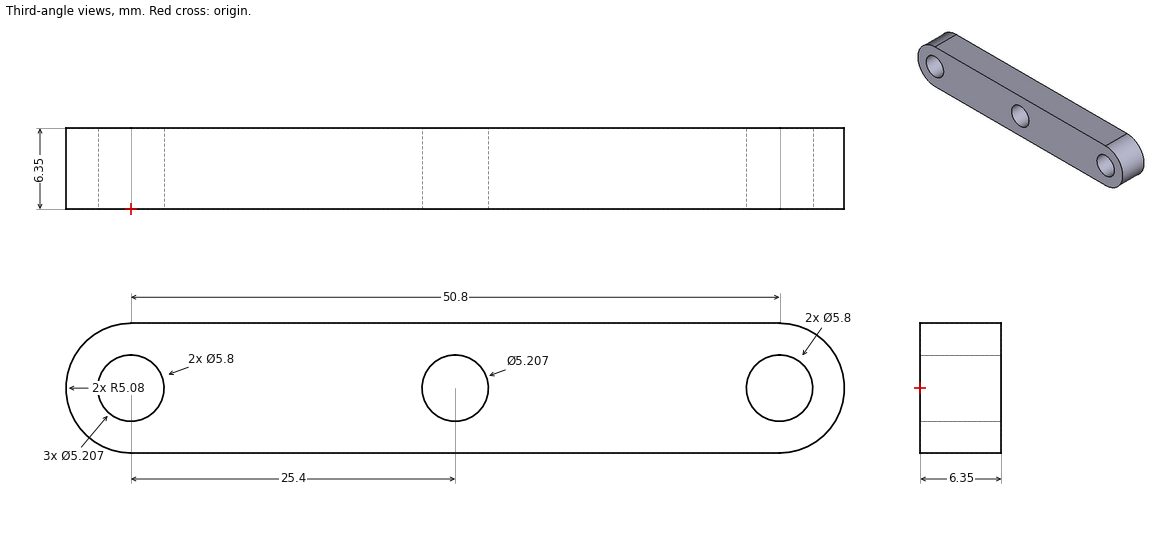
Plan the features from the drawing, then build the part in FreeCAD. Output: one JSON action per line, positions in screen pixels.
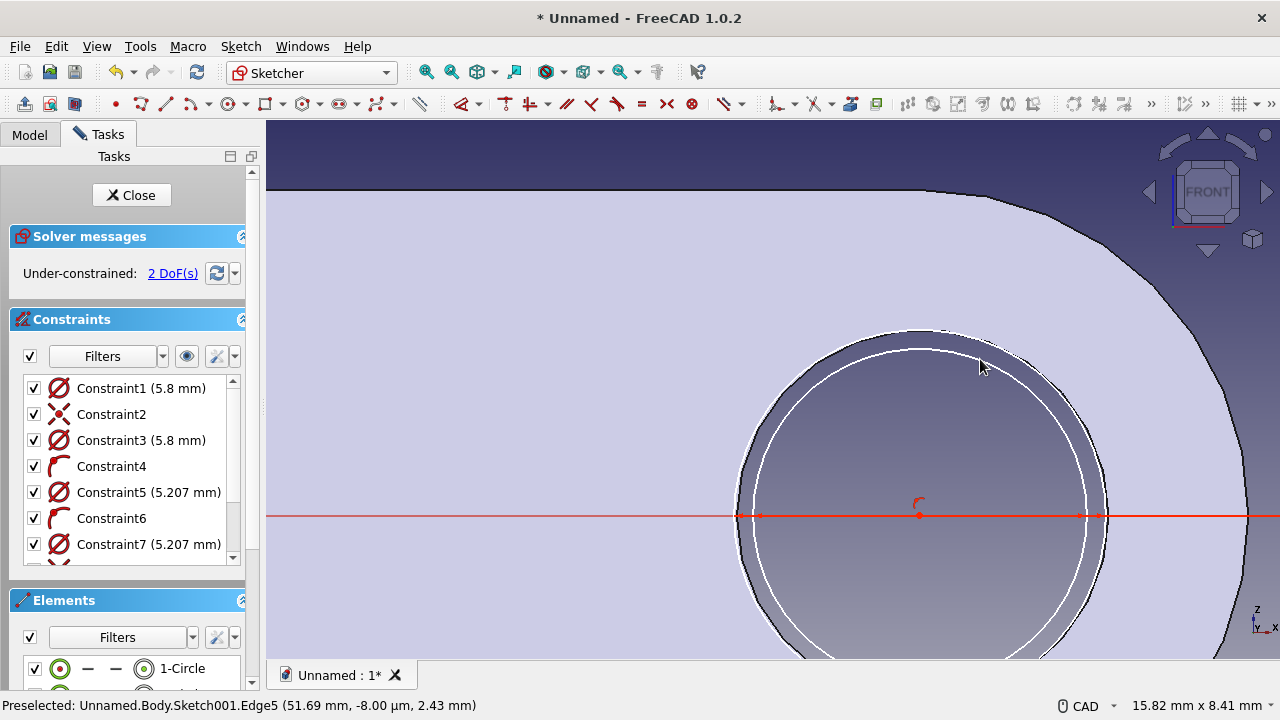
{"action": "key", "text": "d"}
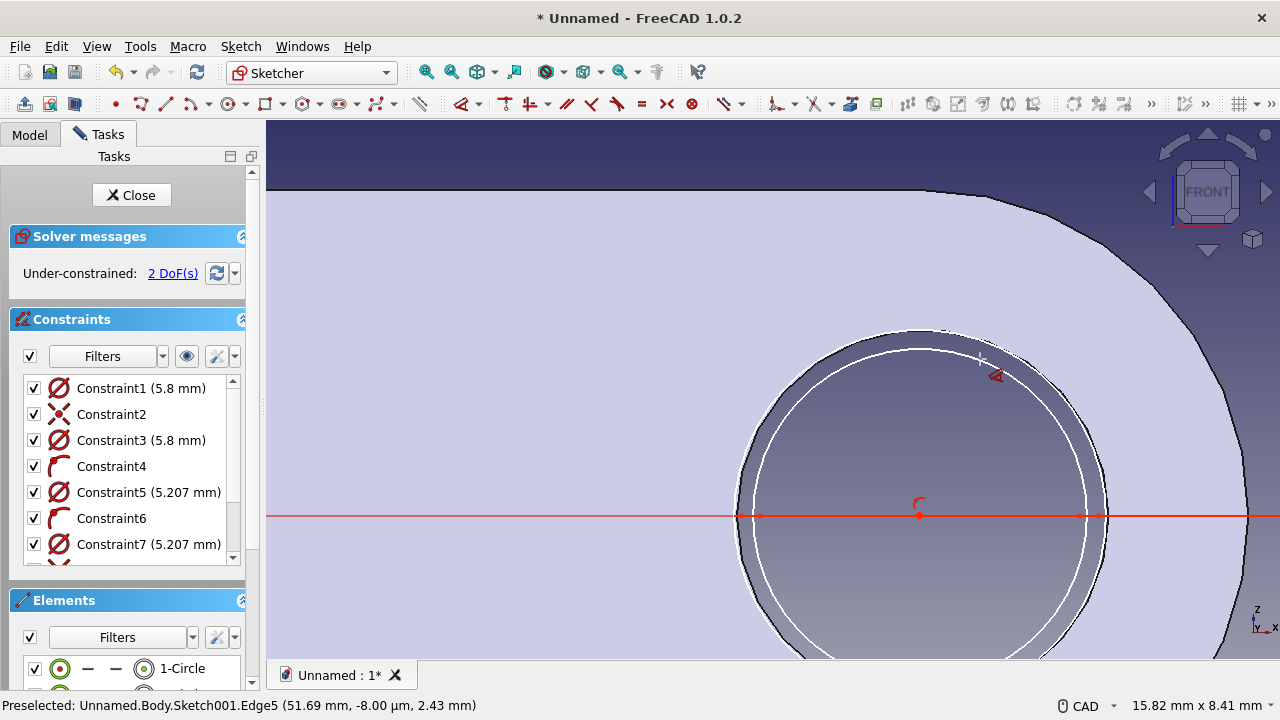
{"action": "scroll", "coordinate": [984, 364], "scroll_direction": "down", "scroll_amount": 9}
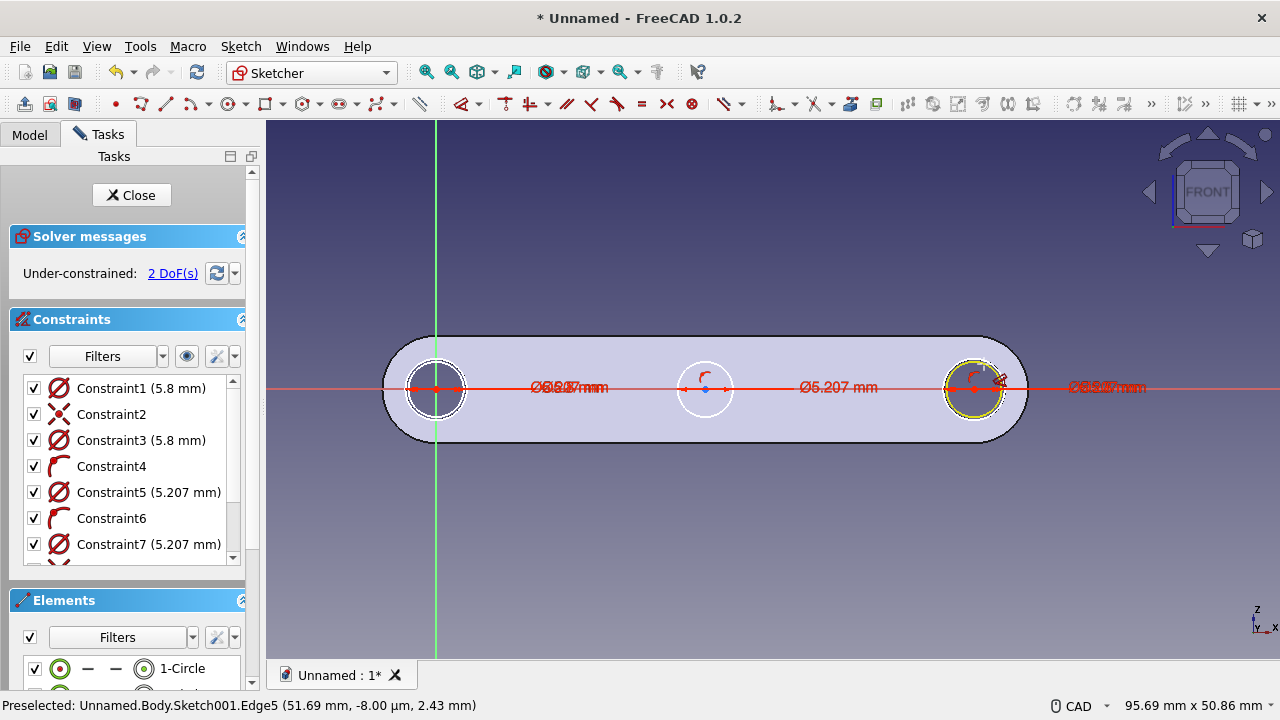
{"action": "left_click", "coordinate": [974, 389]}
{"action": "left_click", "coordinate": [581, 423]}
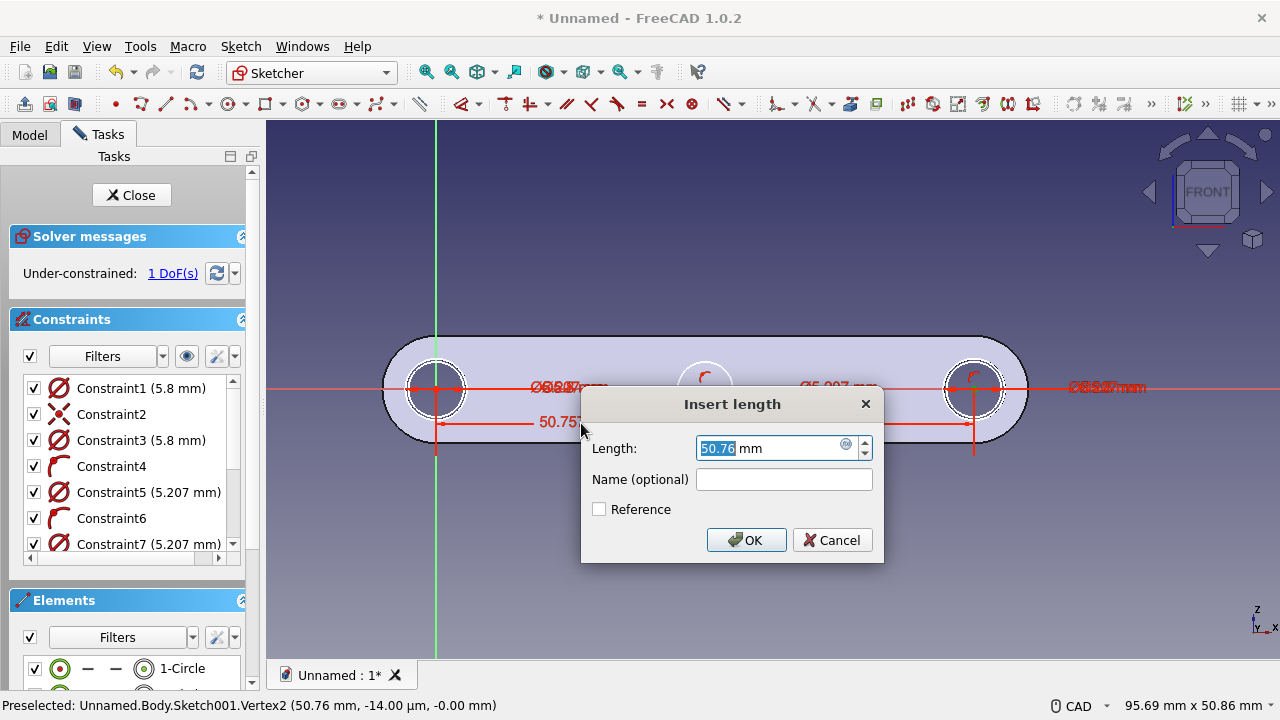
{"action": "type", "text": "50.8"}
{"action": "key", "text": "Return"}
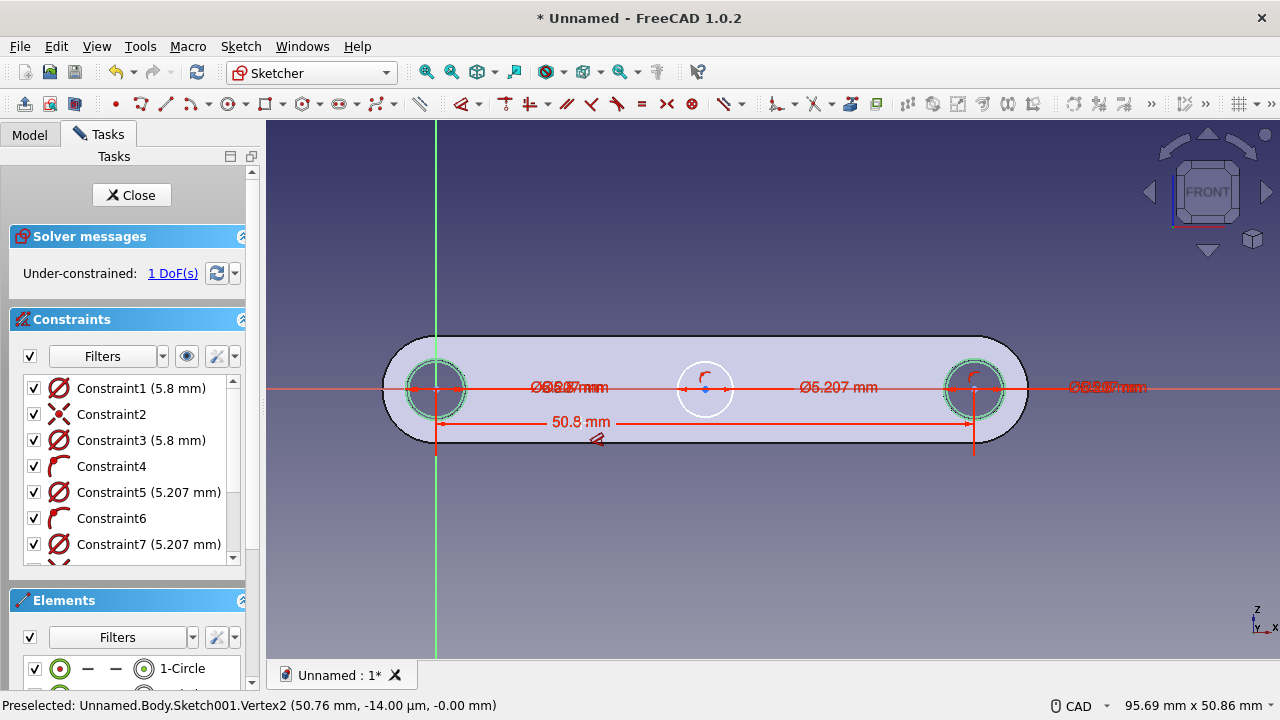
{"action": "left_click", "coordinate": [705, 389]}
{"action": "left_click", "coordinate": [509, 423]}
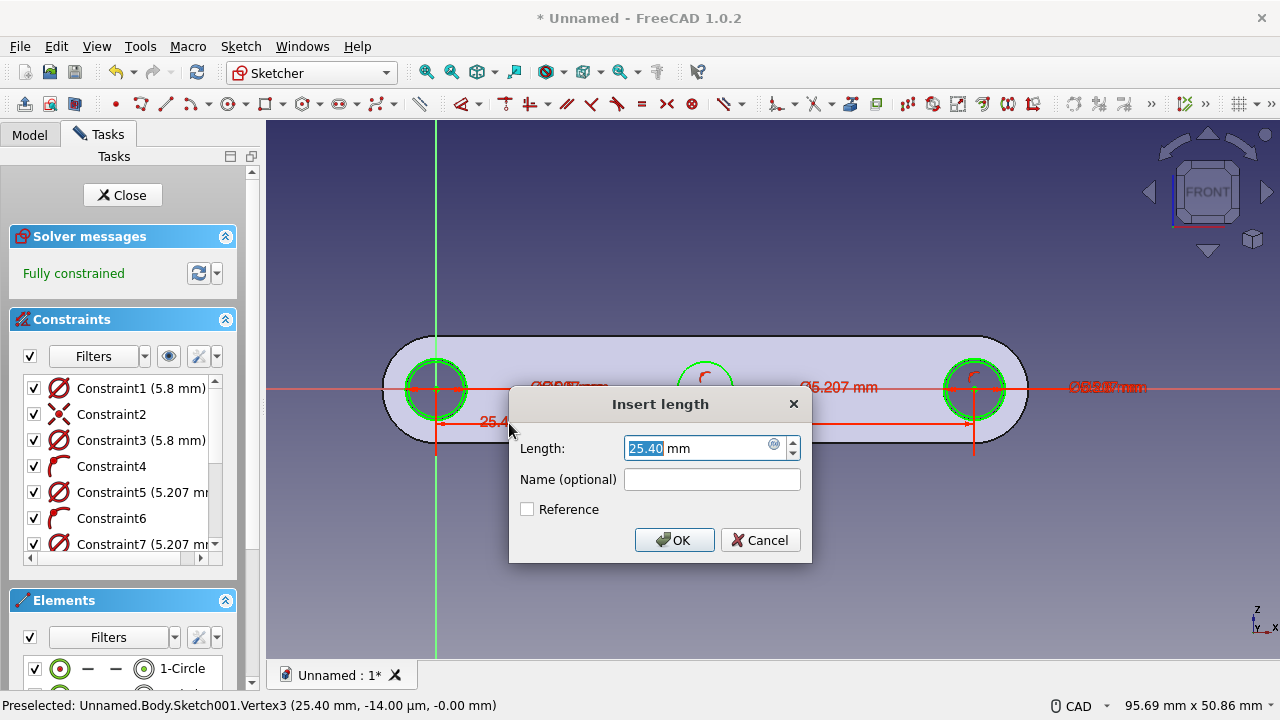
{"action": "type", "text": "25.4"}
{"action": "key", "text": "Return"}
{"action": "key", "text": "Escape"}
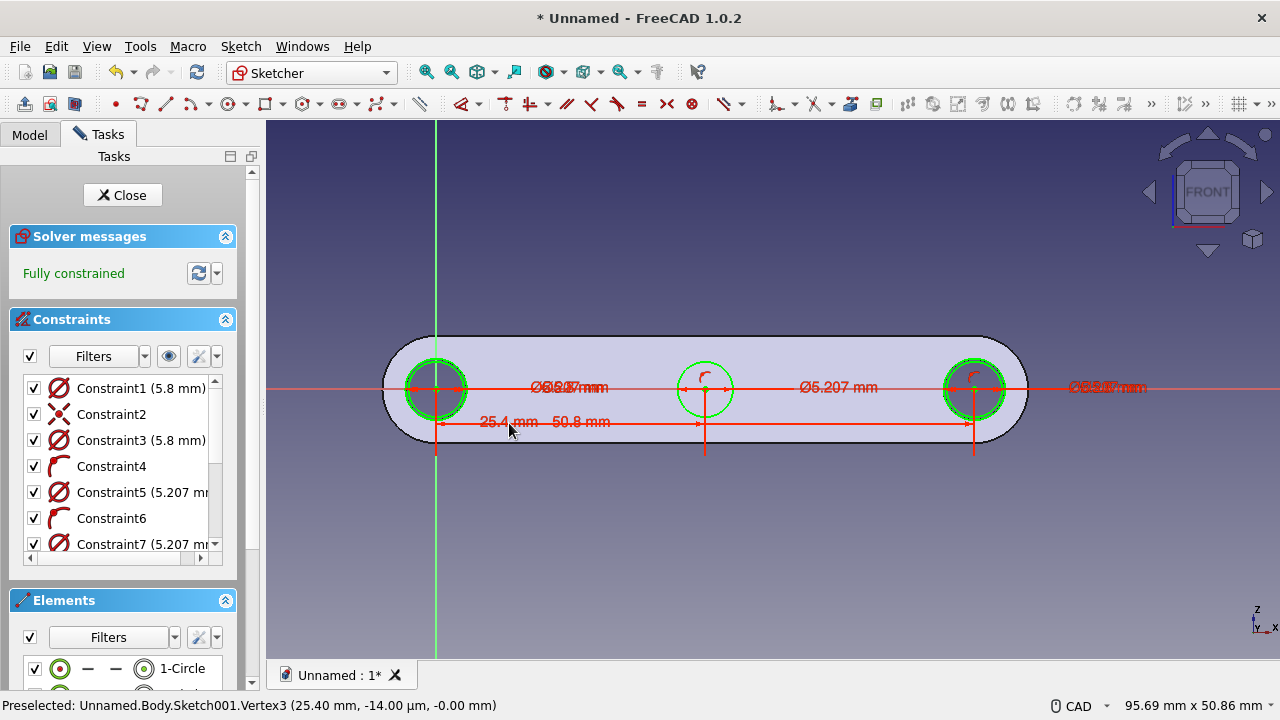
{"action": "left_click", "coordinate": [123, 195]}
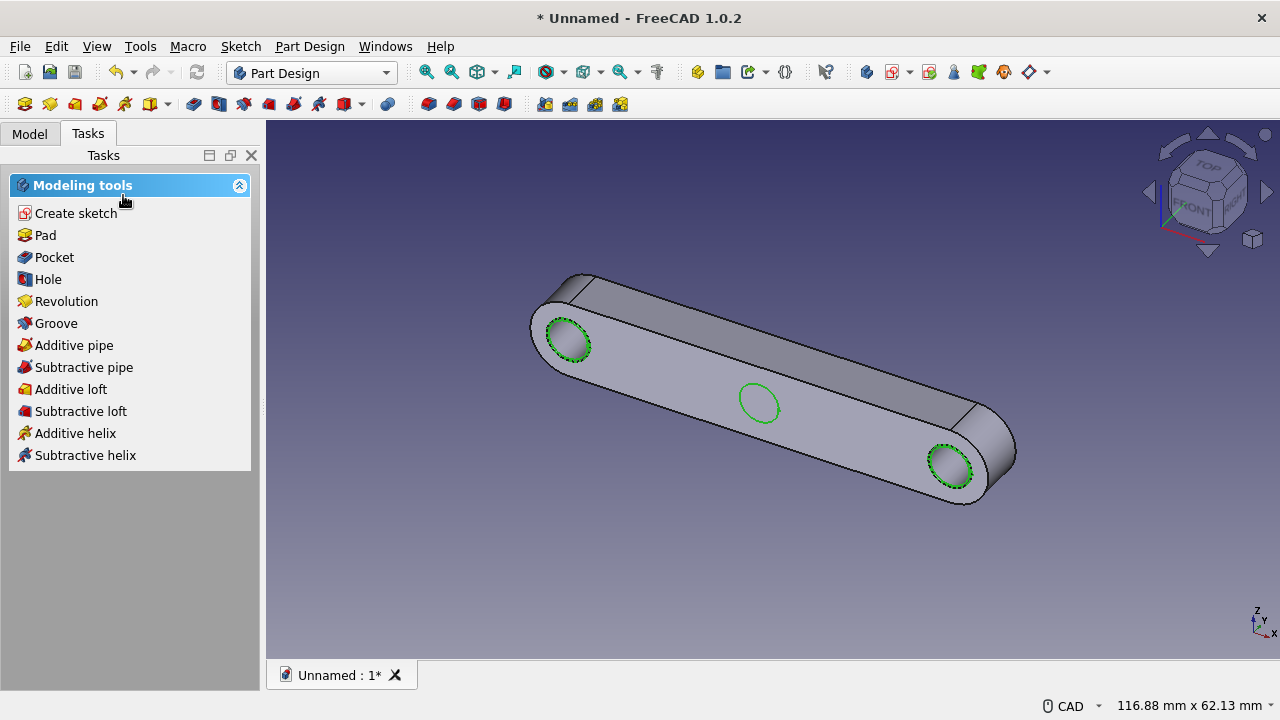
{"action": "left_click", "coordinate": [25, 104]}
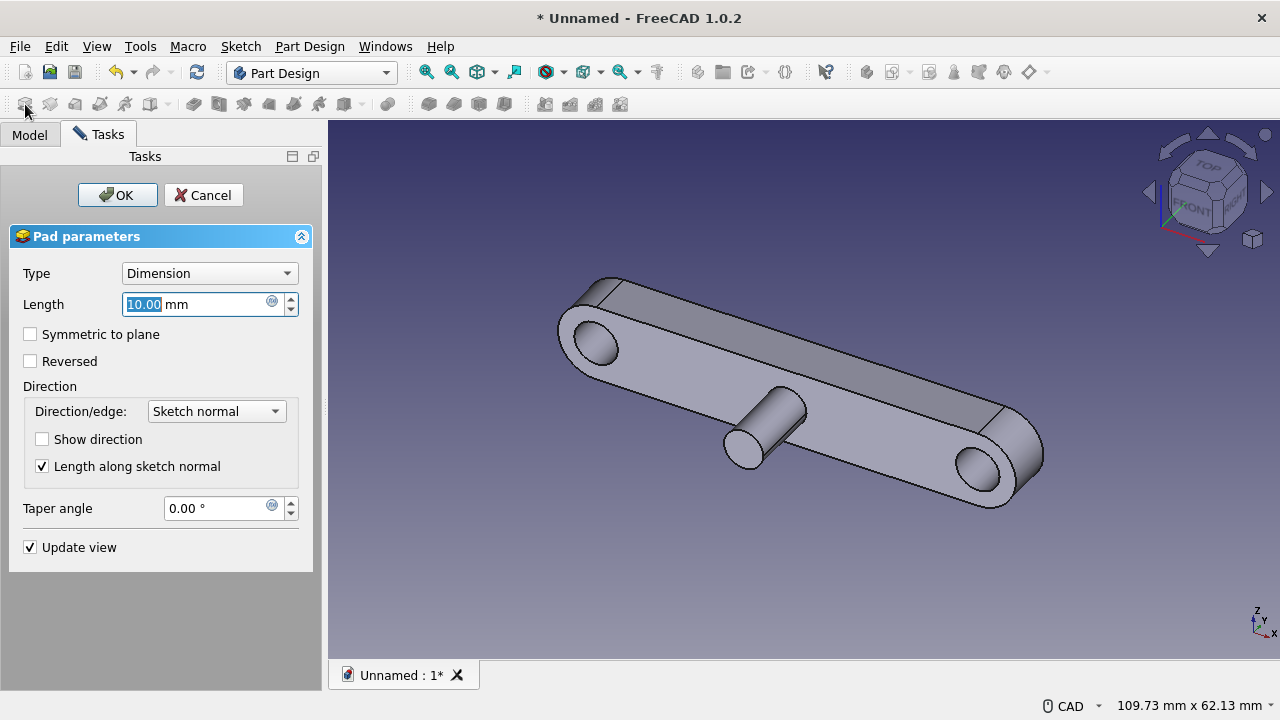
{"action": "type", "text": "6.35"}
{"action": "key", "text": "Tab"}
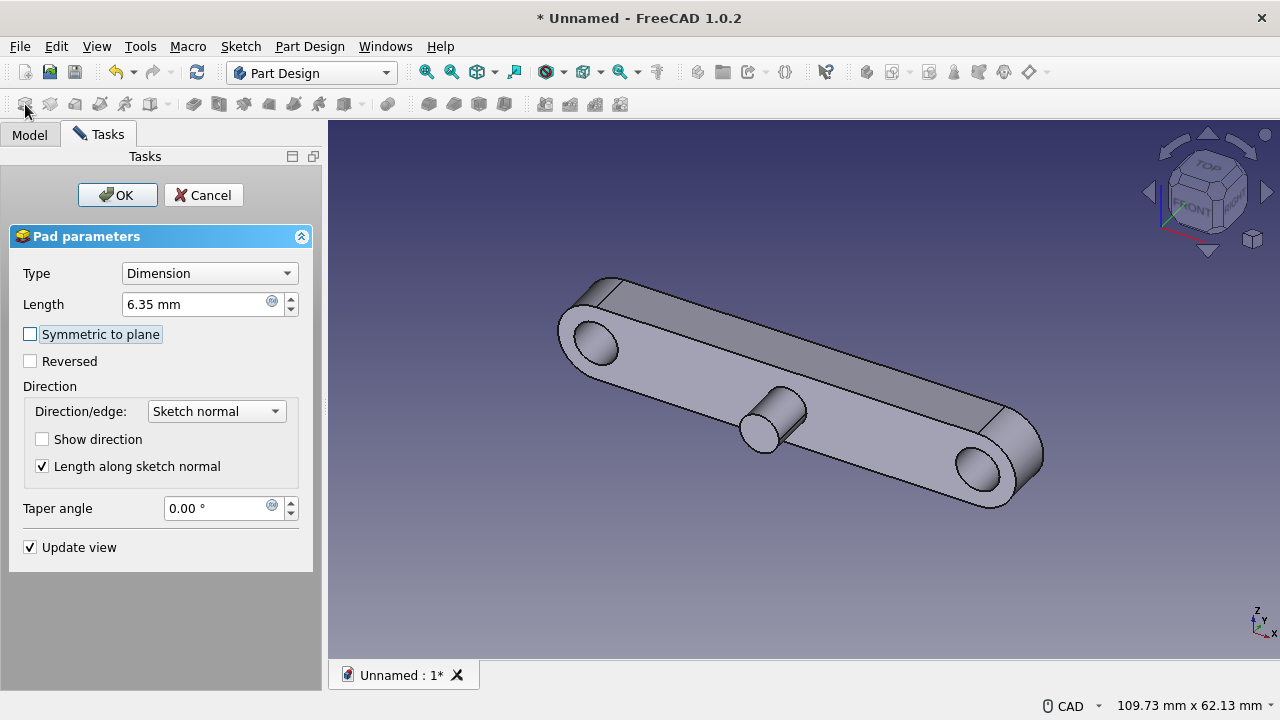
{"action": "left_click", "coordinate": [31, 361]}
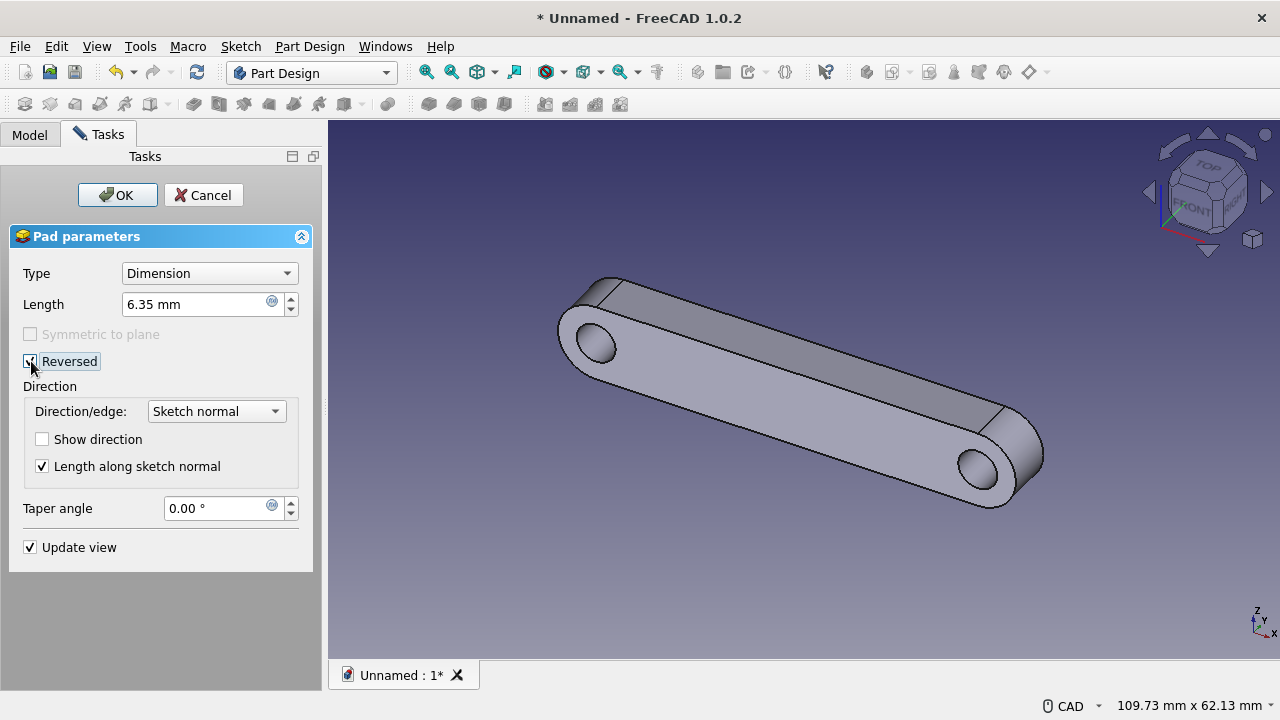
{"action": "left_click", "coordinate": [118, 195]}